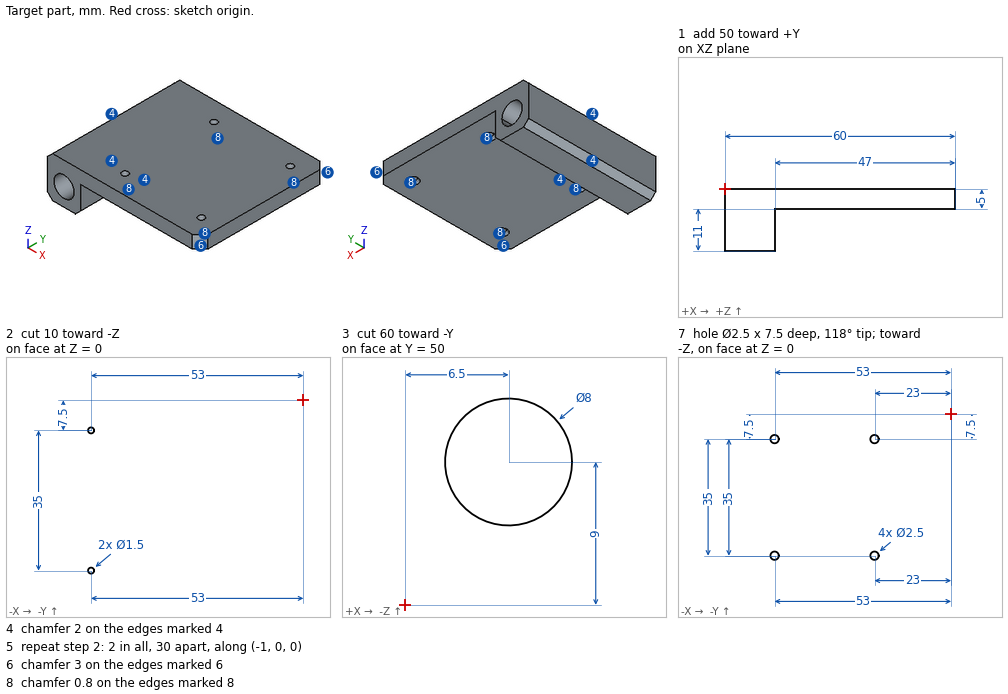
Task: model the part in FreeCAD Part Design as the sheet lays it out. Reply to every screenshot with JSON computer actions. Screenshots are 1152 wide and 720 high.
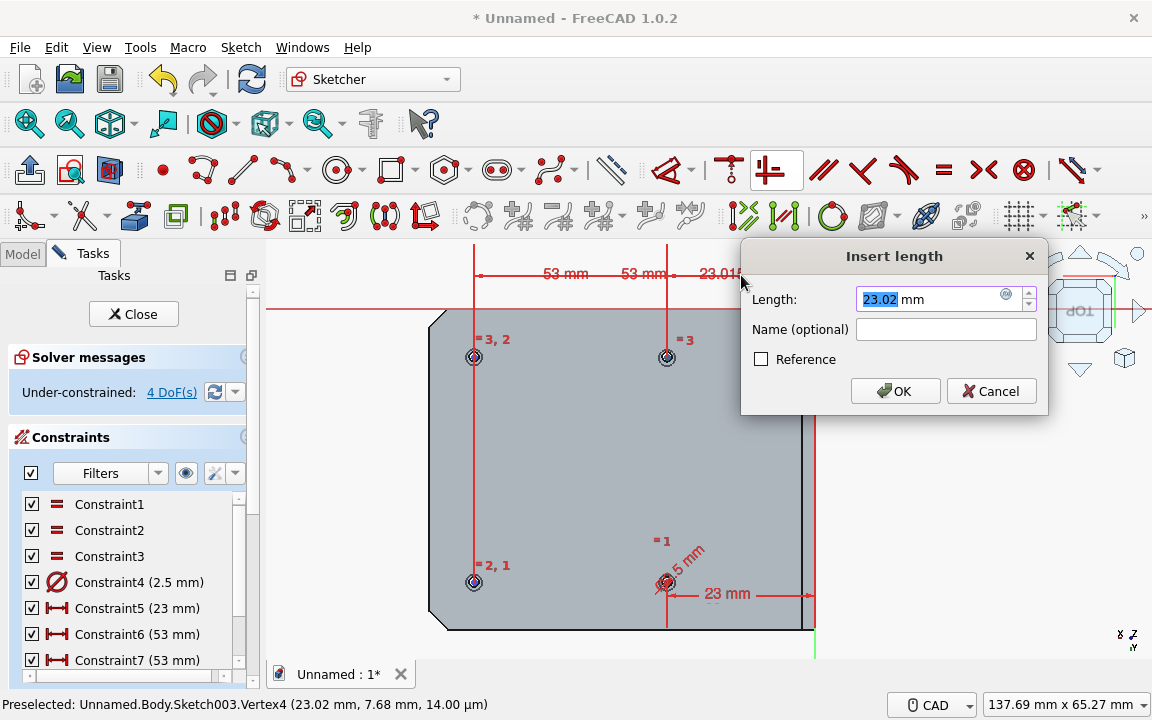
{"action": "type", "text": "23"}
{"action": "key", "text": "Return"}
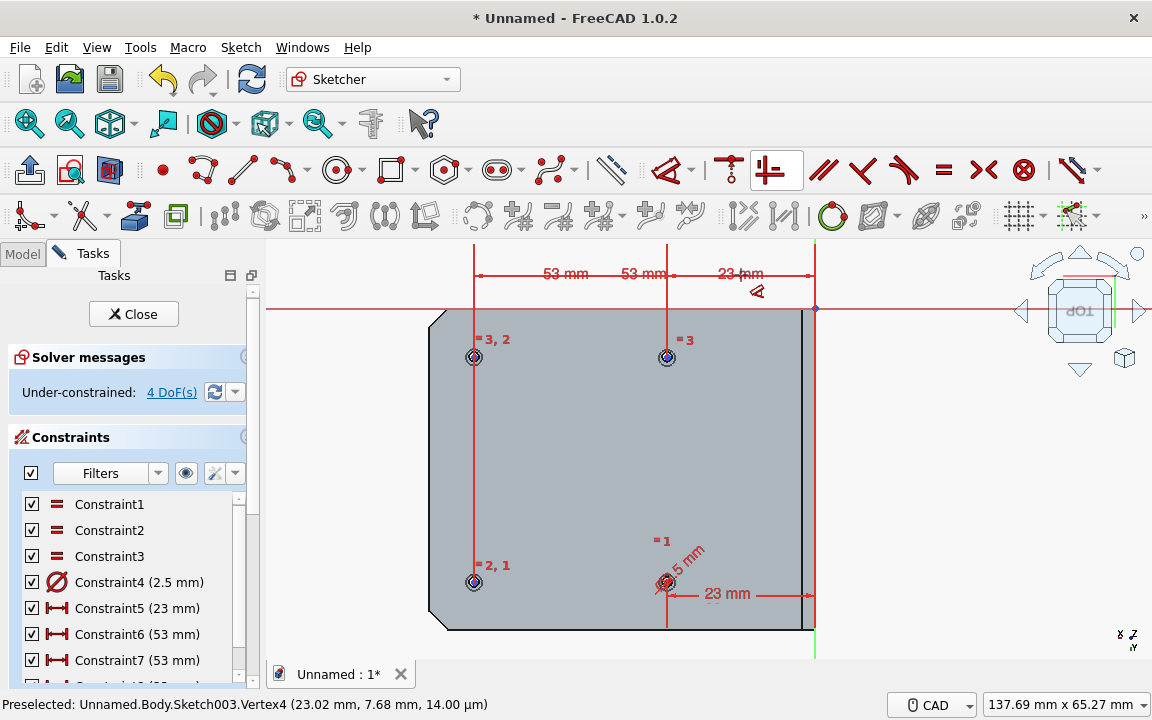
{"action": "left_click", "coordinate": [474, 357]}
{"action": "left_click", "coordinate": [849, 333]}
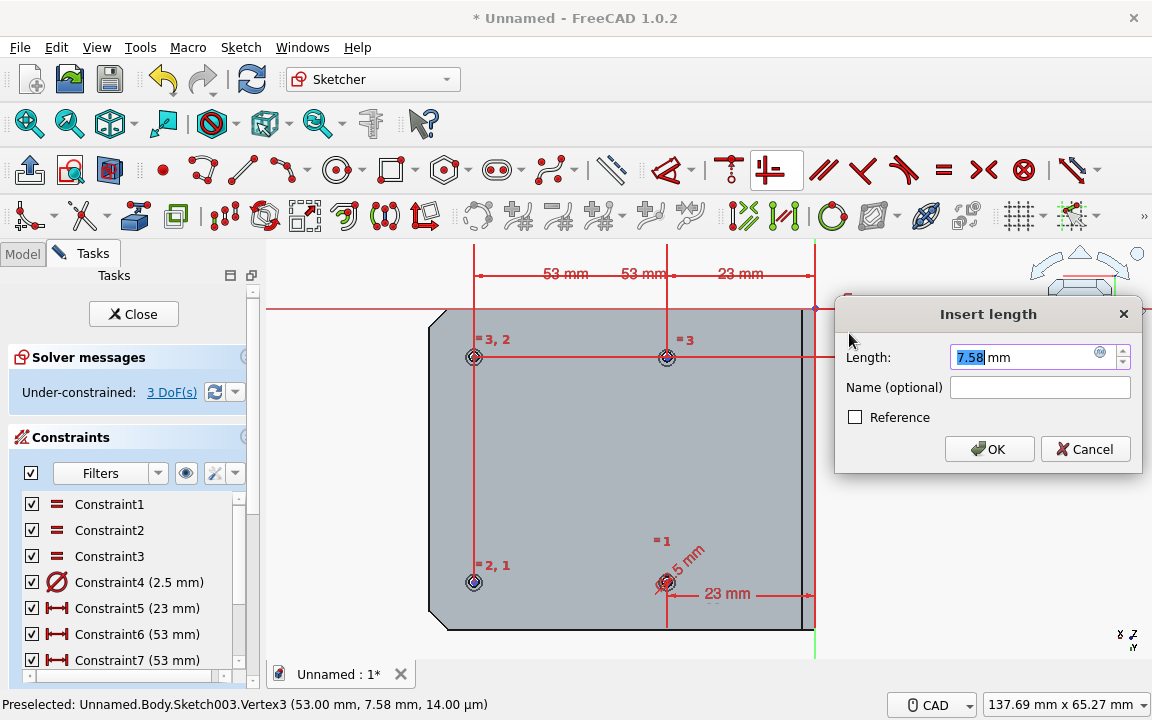
{"action": "type", "text": "7.5"}
{"action": "key", "text": "Return"}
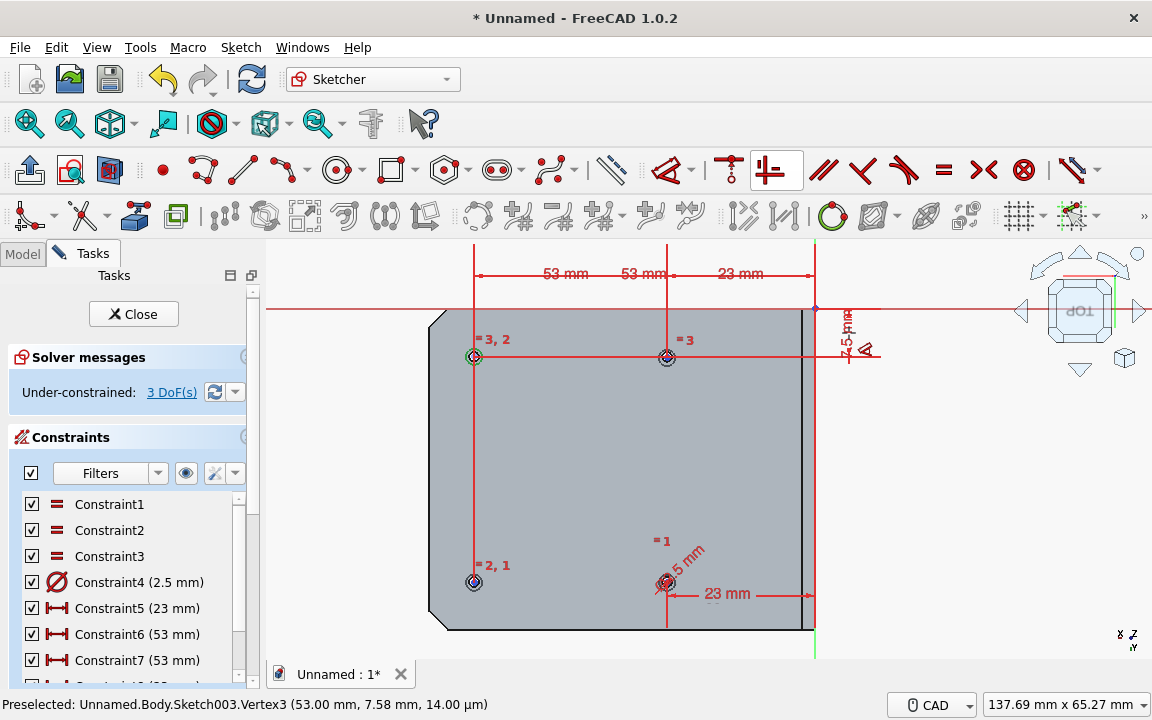
{"action": "left_click", "coordinate": [667, 358]}
{"action": "left_click", "coordinate": [633, 333]}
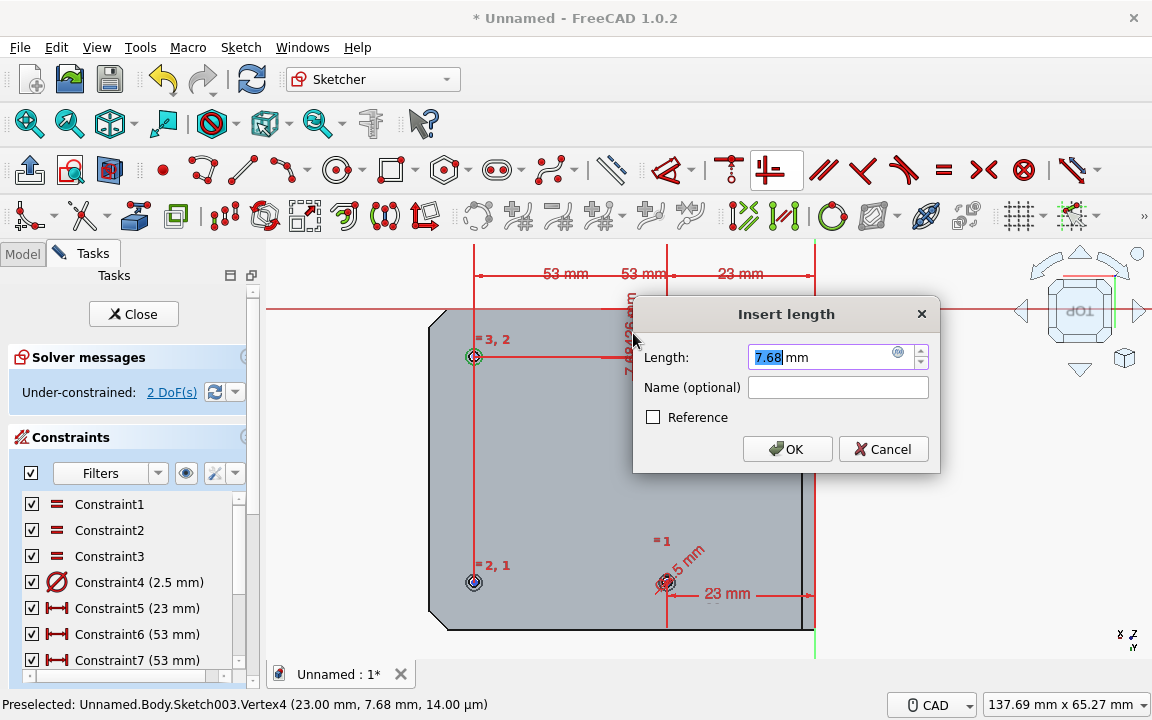
{"action": "type", "text": "7.5"}
{"action": "key", "text": "Return"}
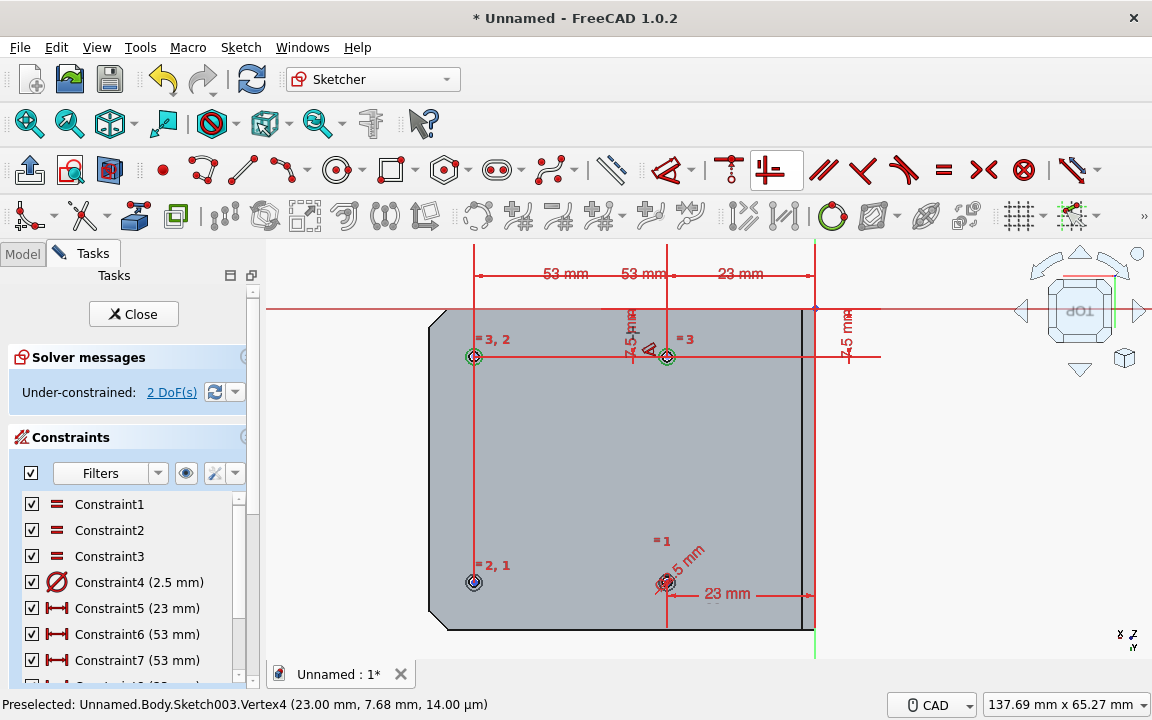
{"action": "left_click", "coordinate": [474, 583]}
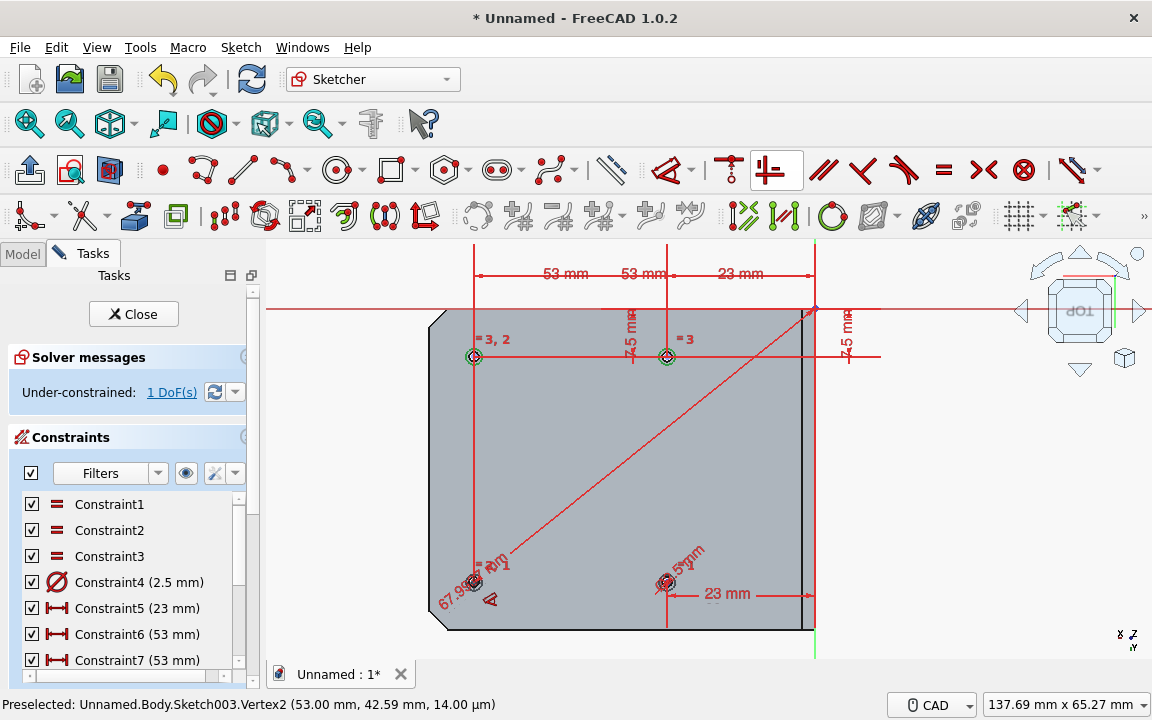
{"action": "left_click", "coordinate": [474, 357]}
{"action": "left_click", "coordinate": [440, 470]}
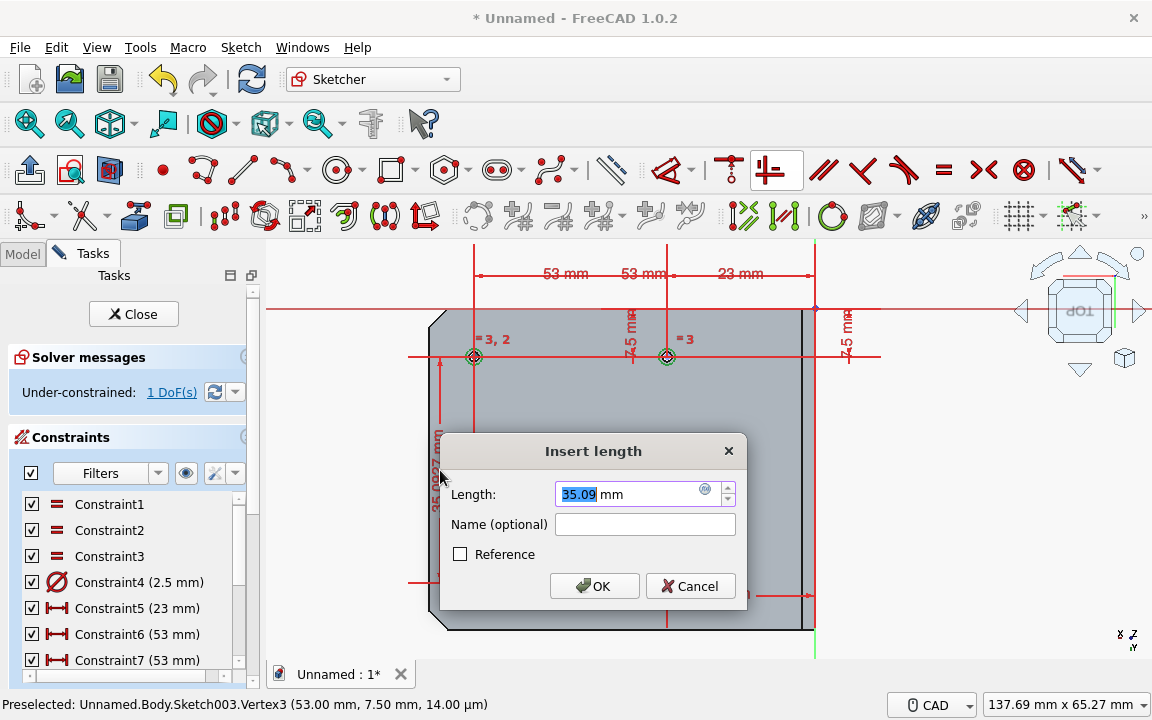
{"action": "type", "text": "35"}
{"action": "key", "text": "Return"}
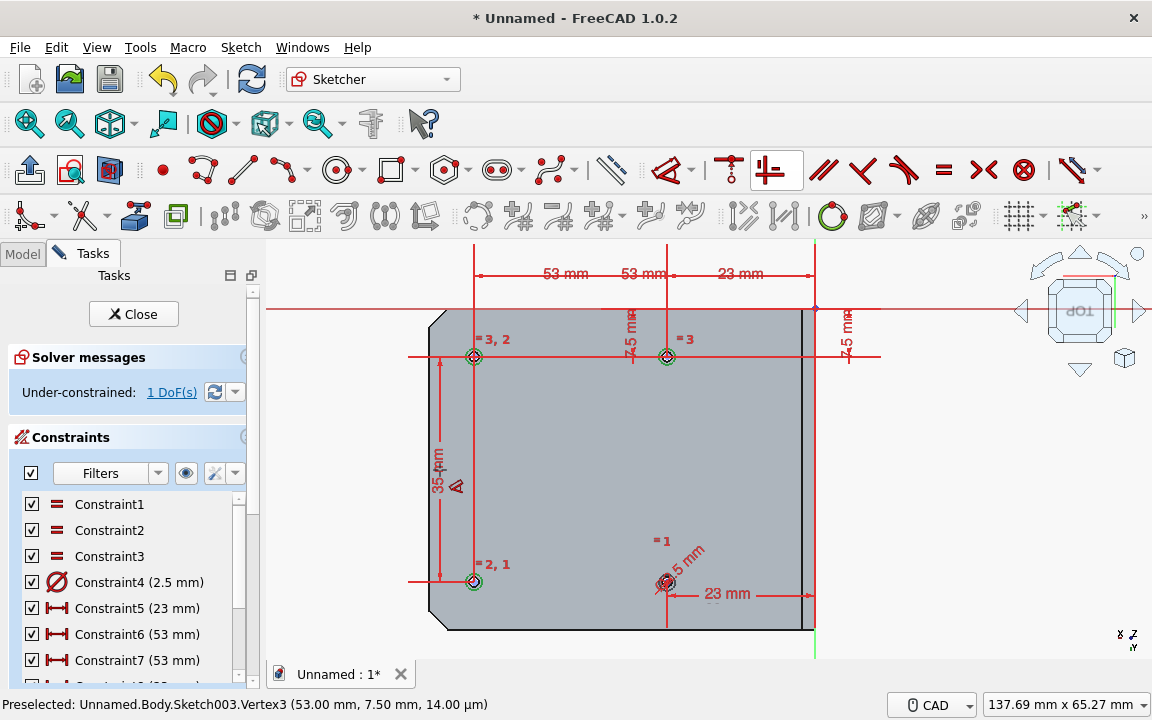
{"action": "left_click", "coordinate": [667, 583]}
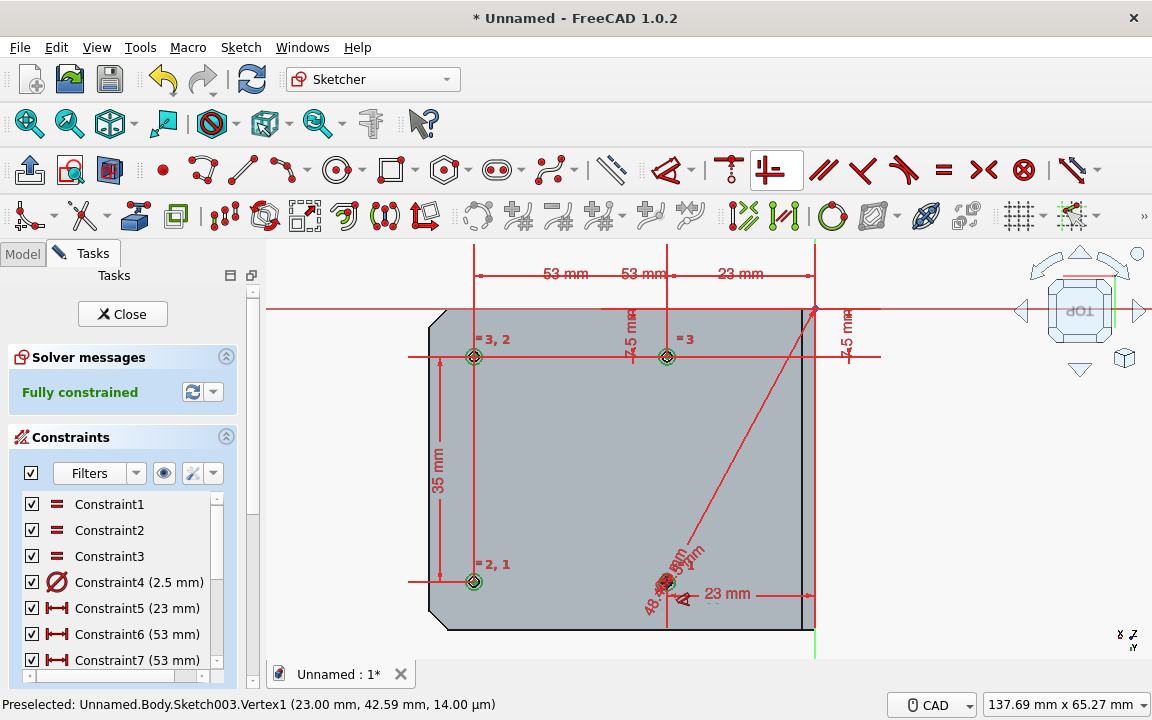
{"action": "left_click", "coordinate": [474, 357]}
{"action": "left_click", "coordinate": [440, 418]}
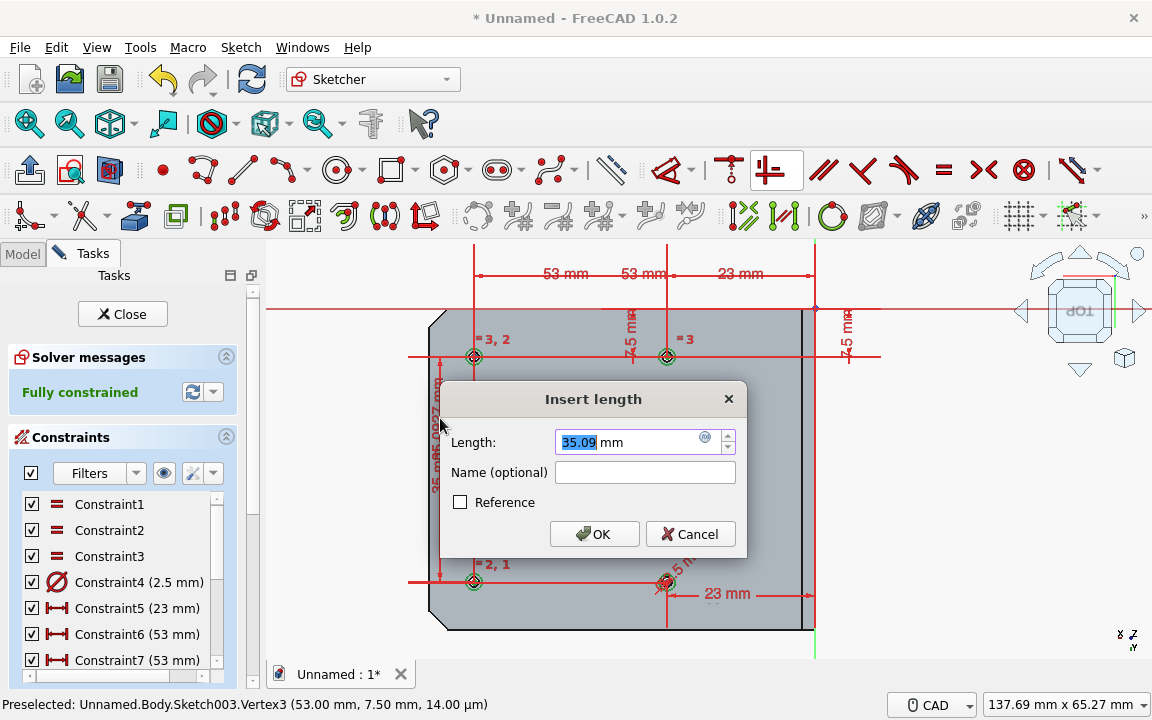
{"action": "type", "text": "35"}
{"action": "key", "text": "Return"}
{"action": "key", "text": "Escape"}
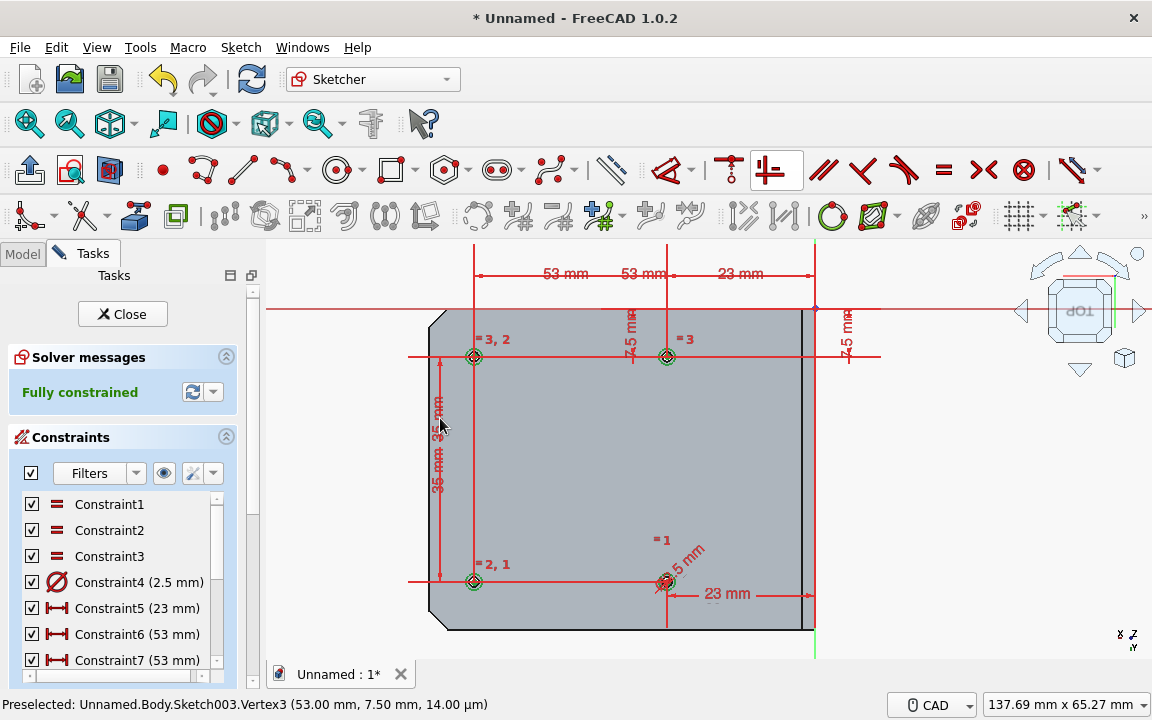
{"action": "left_click", "coordinate": [123, 314]}